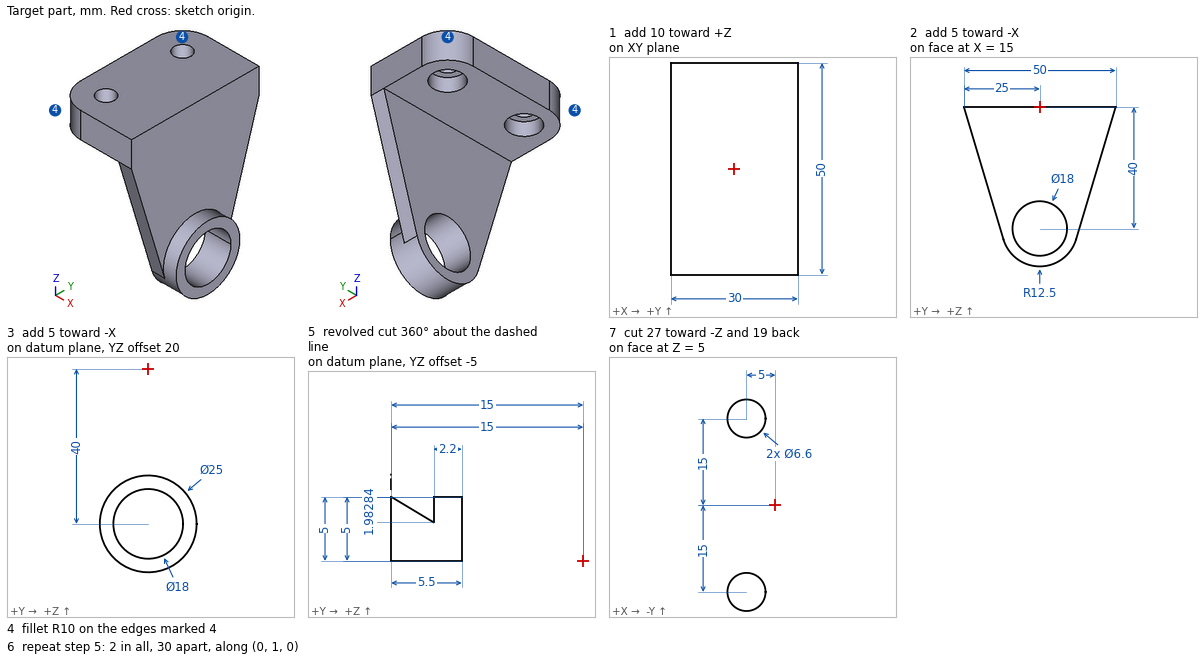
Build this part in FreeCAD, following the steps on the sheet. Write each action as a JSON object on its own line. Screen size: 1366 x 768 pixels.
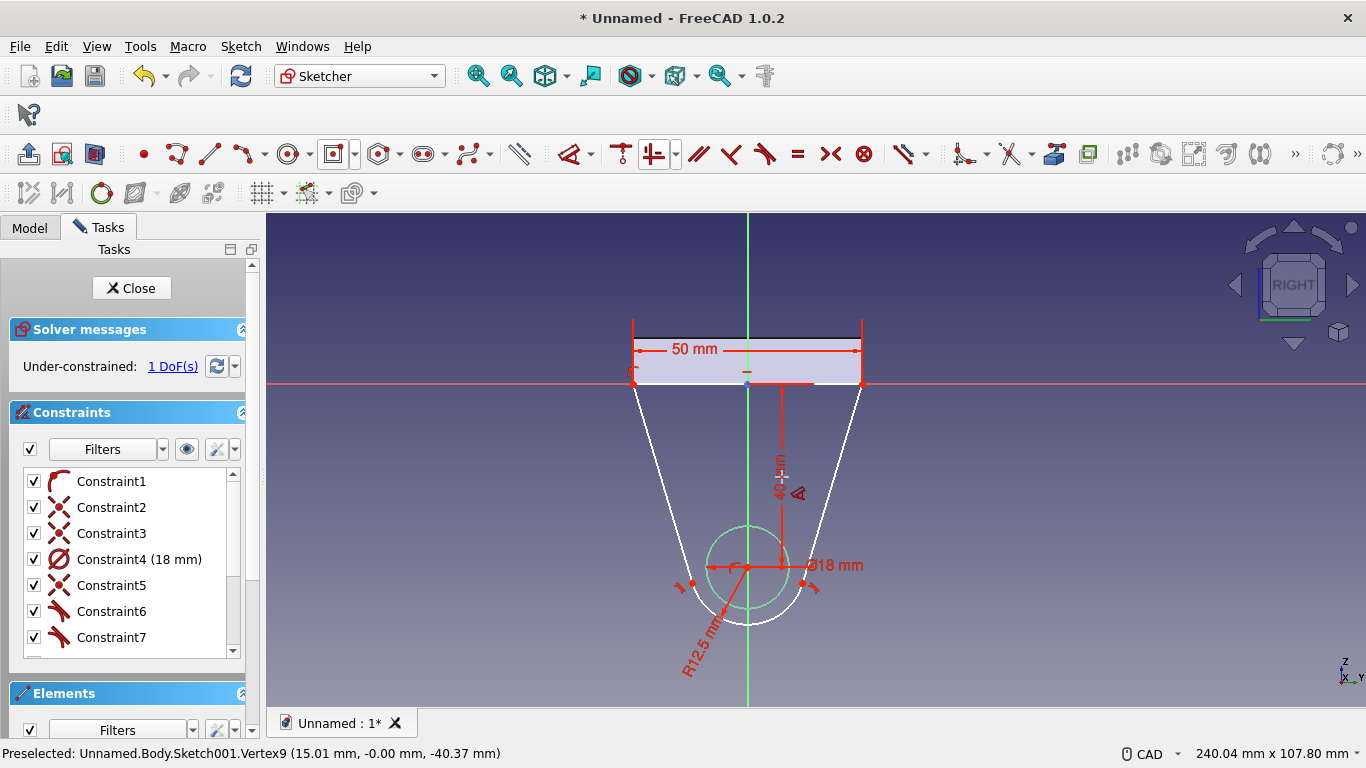
{"action": "left_click", "coordinate": [633, 384]}
{"action": "left_click", "coordinate": [690, 418]}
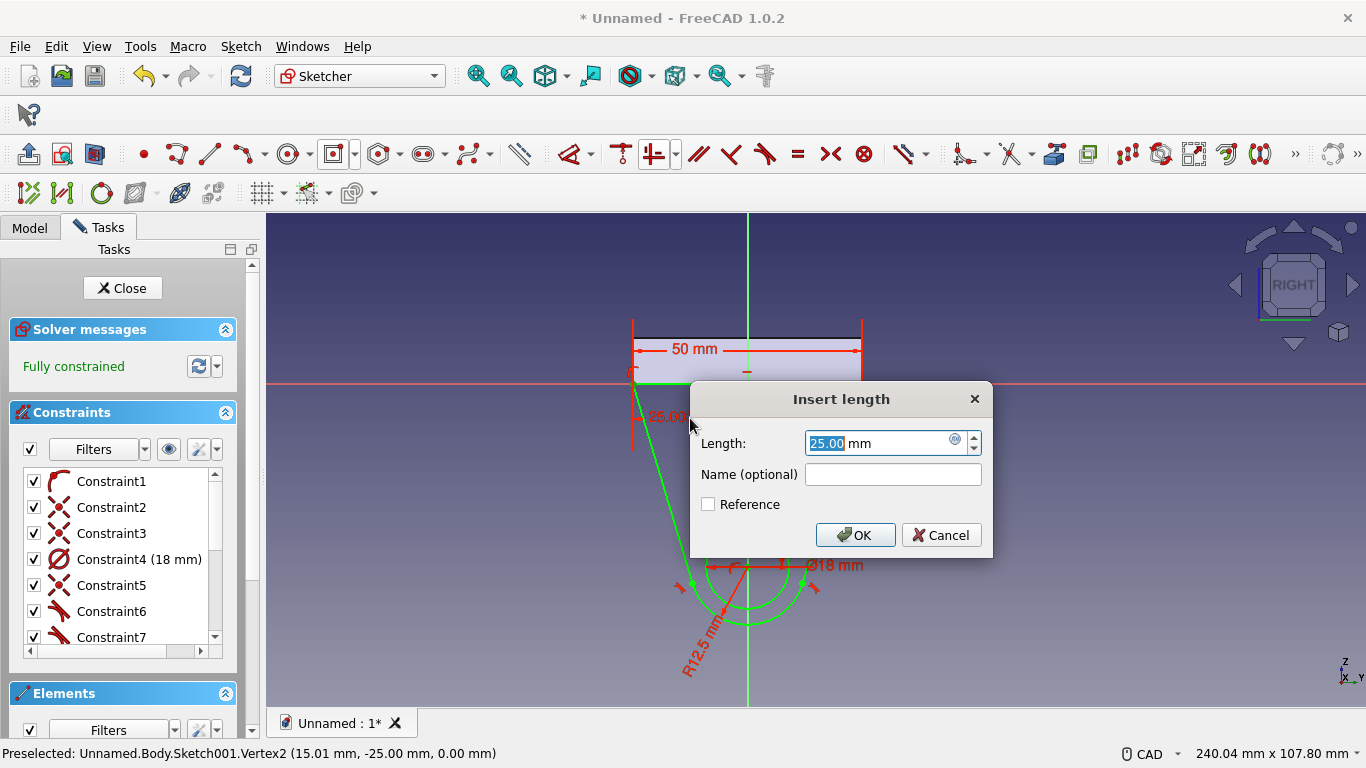
{"action": "type", "text": "25"}
{"action": "key", "text": "Return"}
{"action": "key", "text": "Escape"}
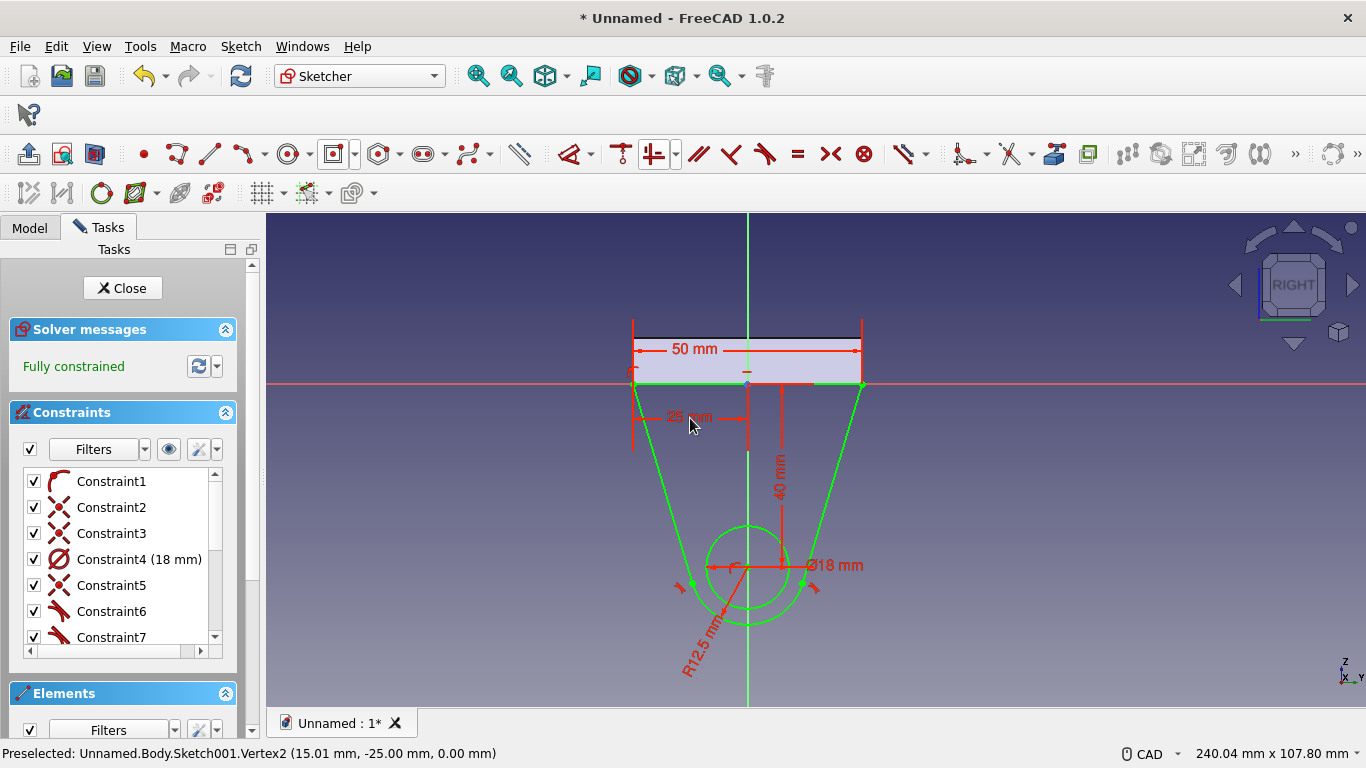
{"action": "left_click", "coordinate": [123, 288]}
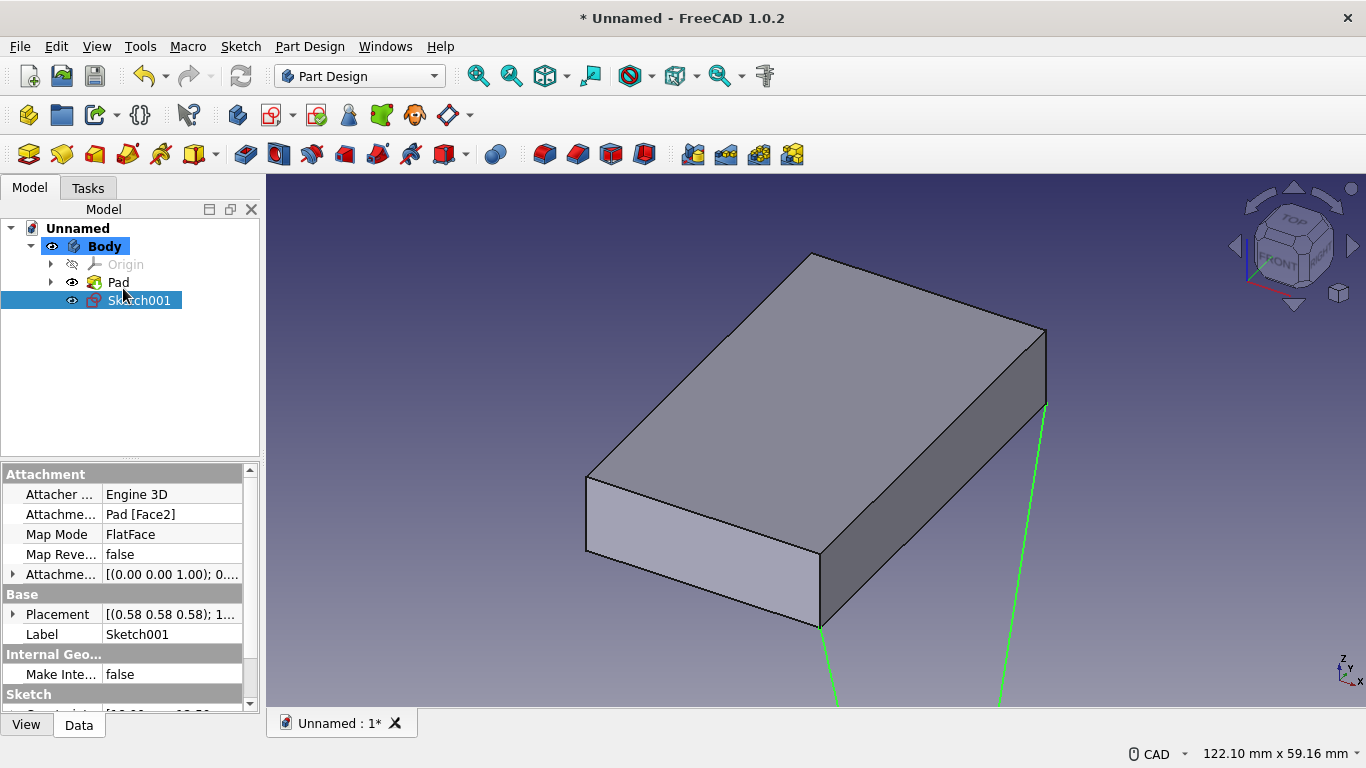
{"action": "left_click", "coordinate": [29, 154]}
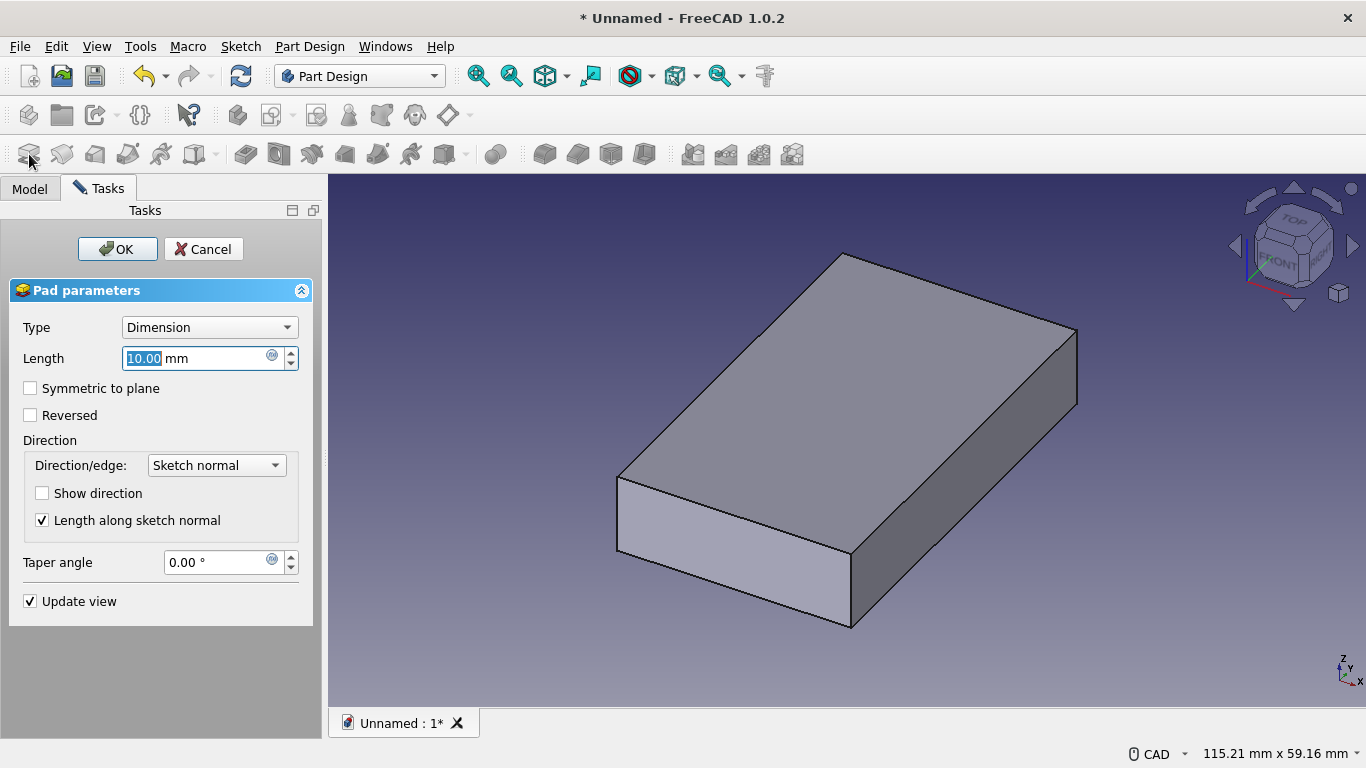
{"action": "type", "text": "5"}
{"action": "key", "text": "Tab"}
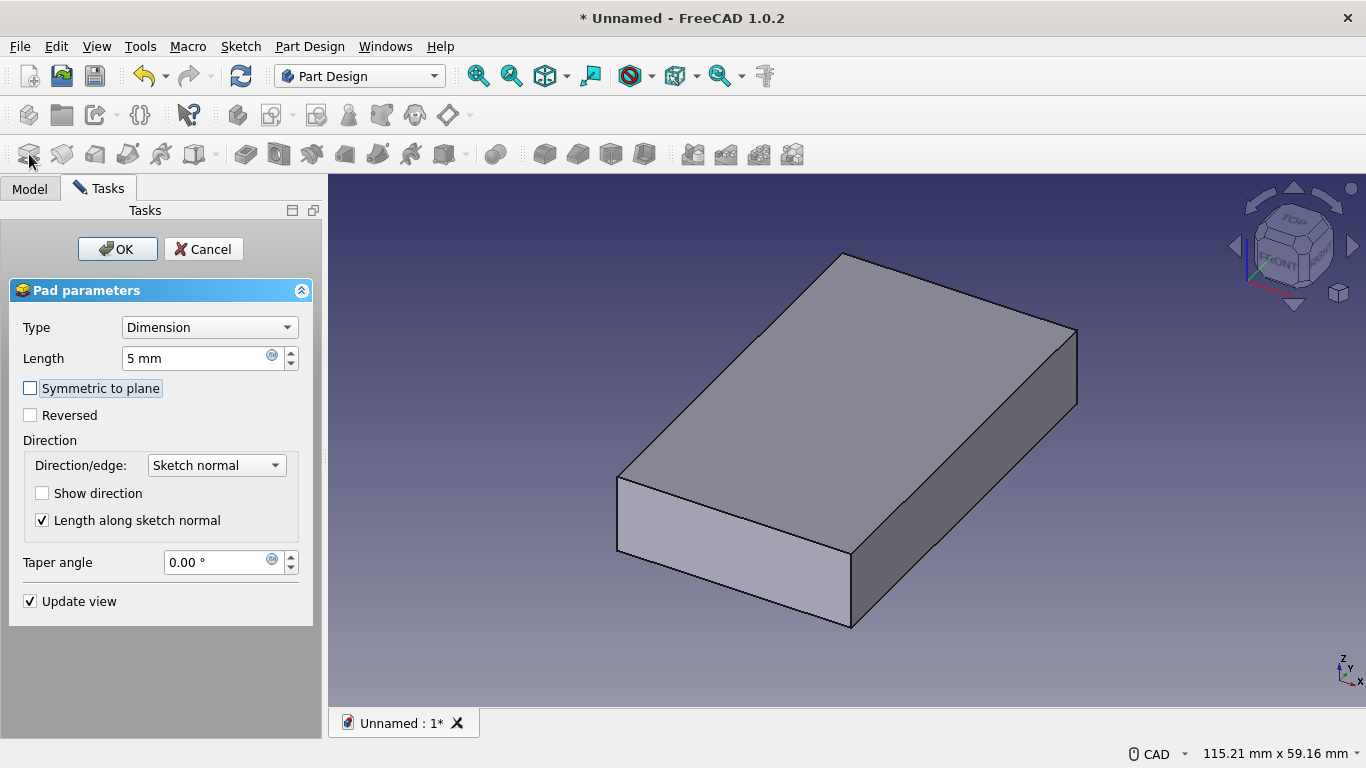
{"action": "left_click", "coordinate": [31, 415]}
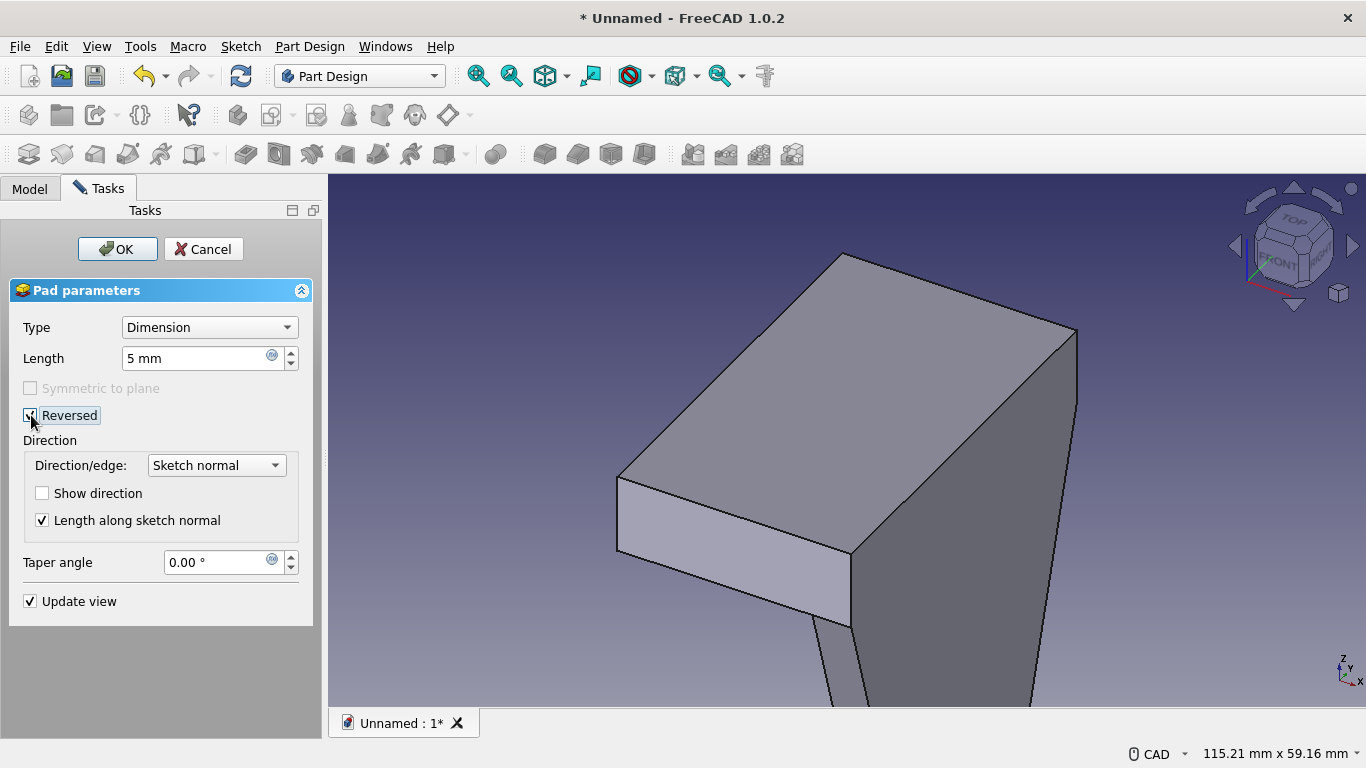
{"action": "left_click", "coordinate": [118, 249]}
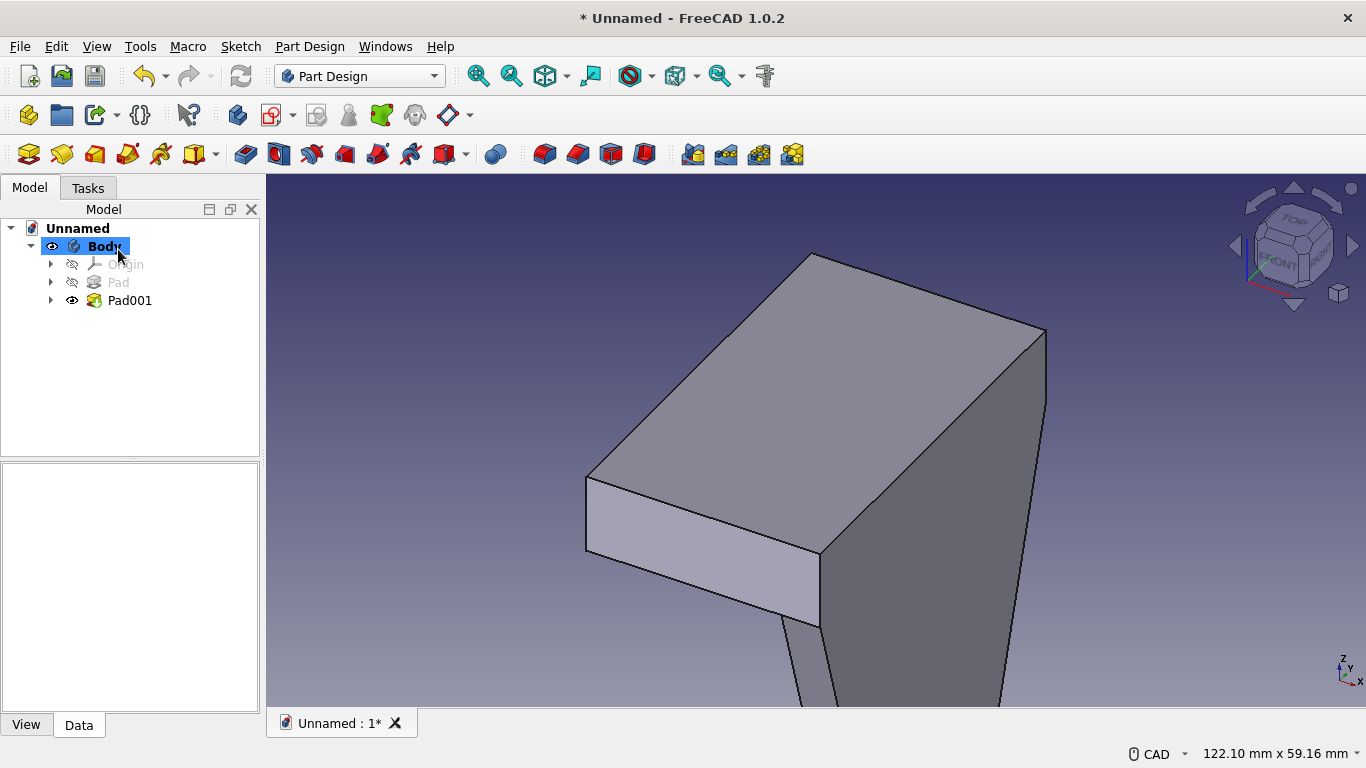
{"action": "left_click", "coordinate": [479, 76]}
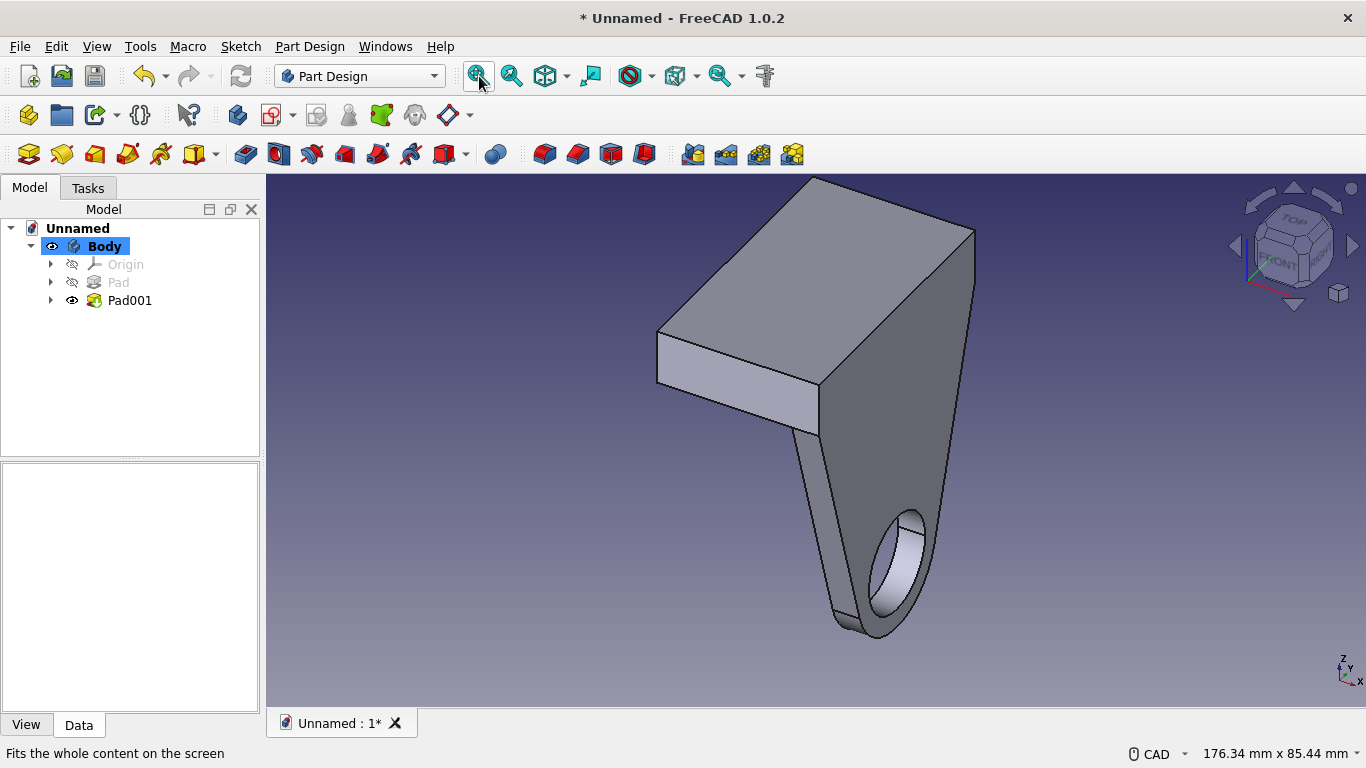
{"action": "left_click", "coordinate": [51, 264]}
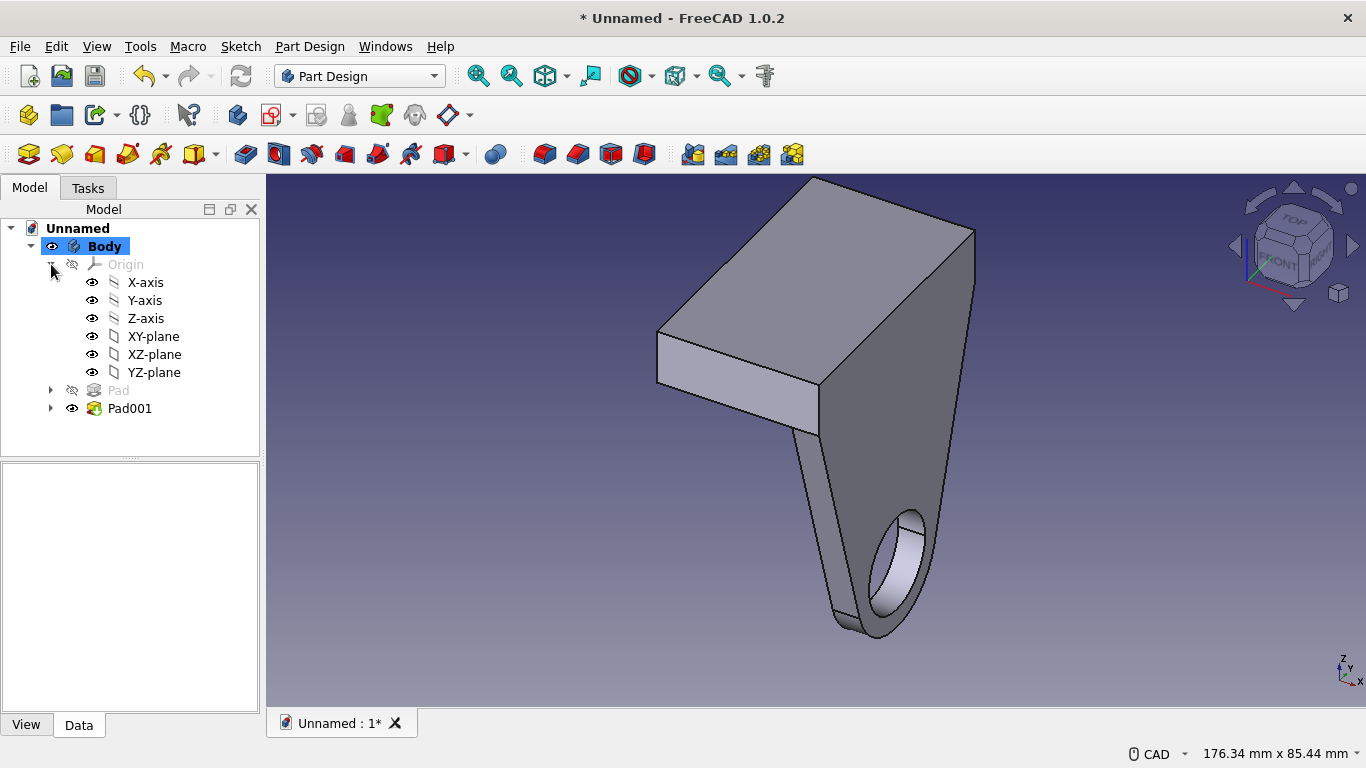
{"action": "left_click", "coordinate": [137, 372]}